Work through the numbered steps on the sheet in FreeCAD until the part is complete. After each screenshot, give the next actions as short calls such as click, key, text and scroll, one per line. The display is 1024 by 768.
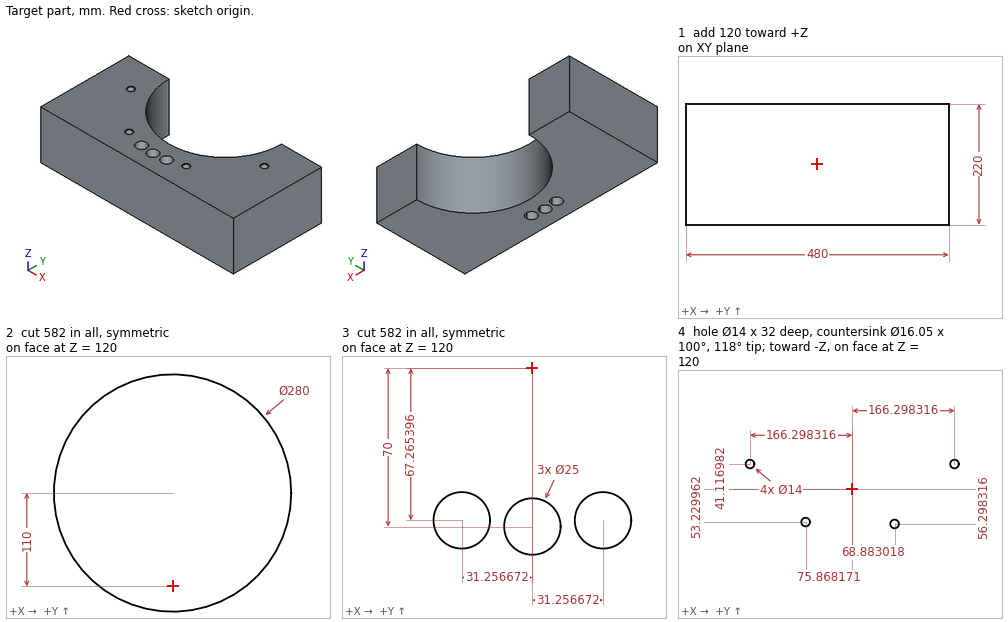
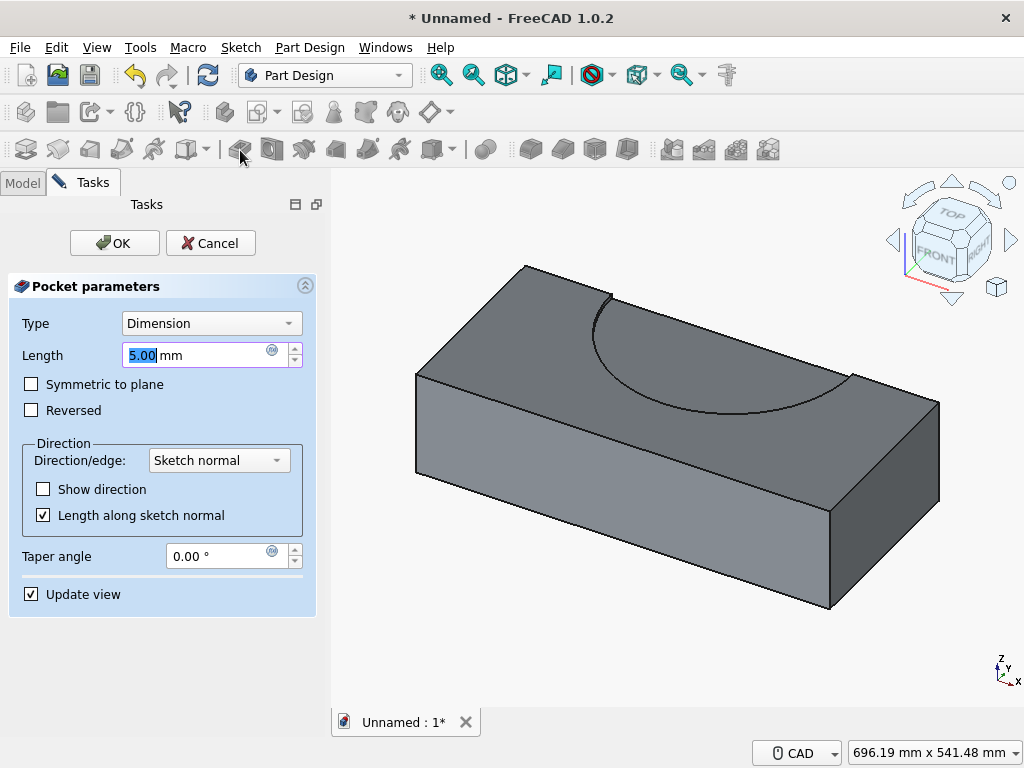
text(582)
key(Tab)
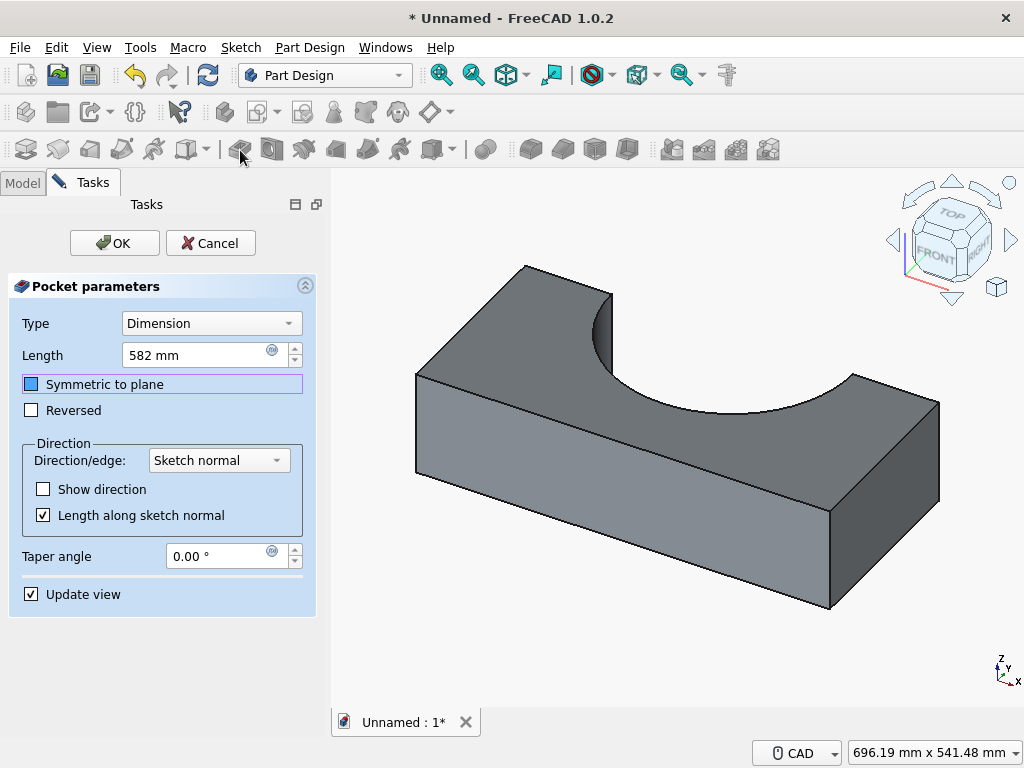
click(30, 384)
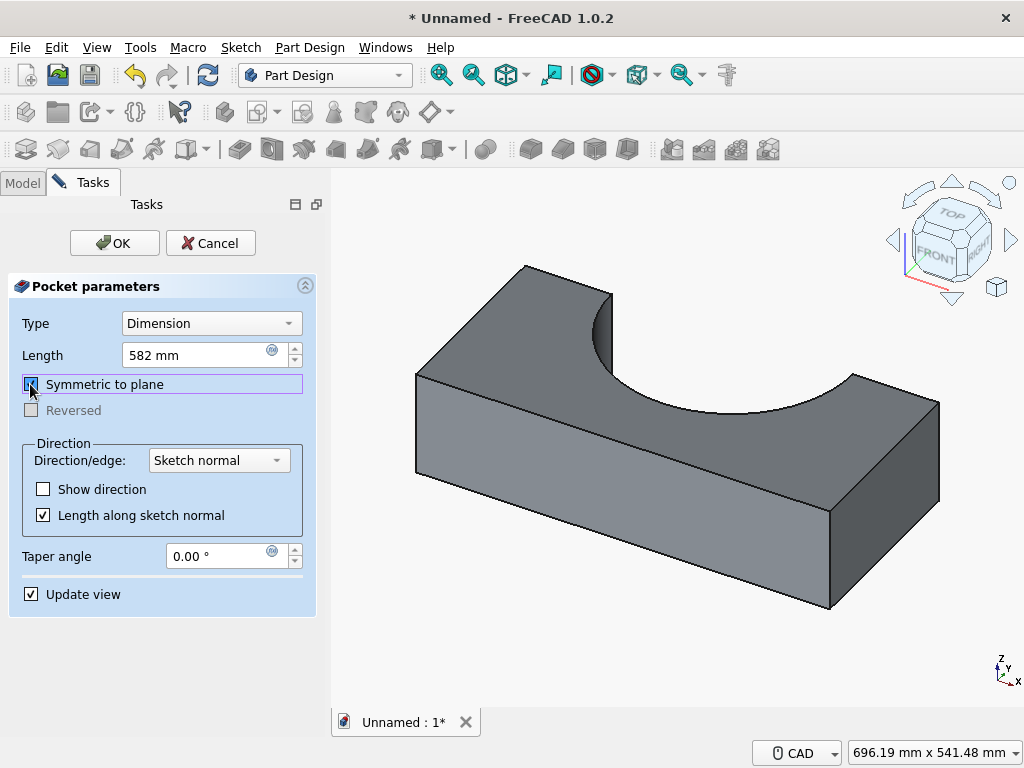
click(115, 243)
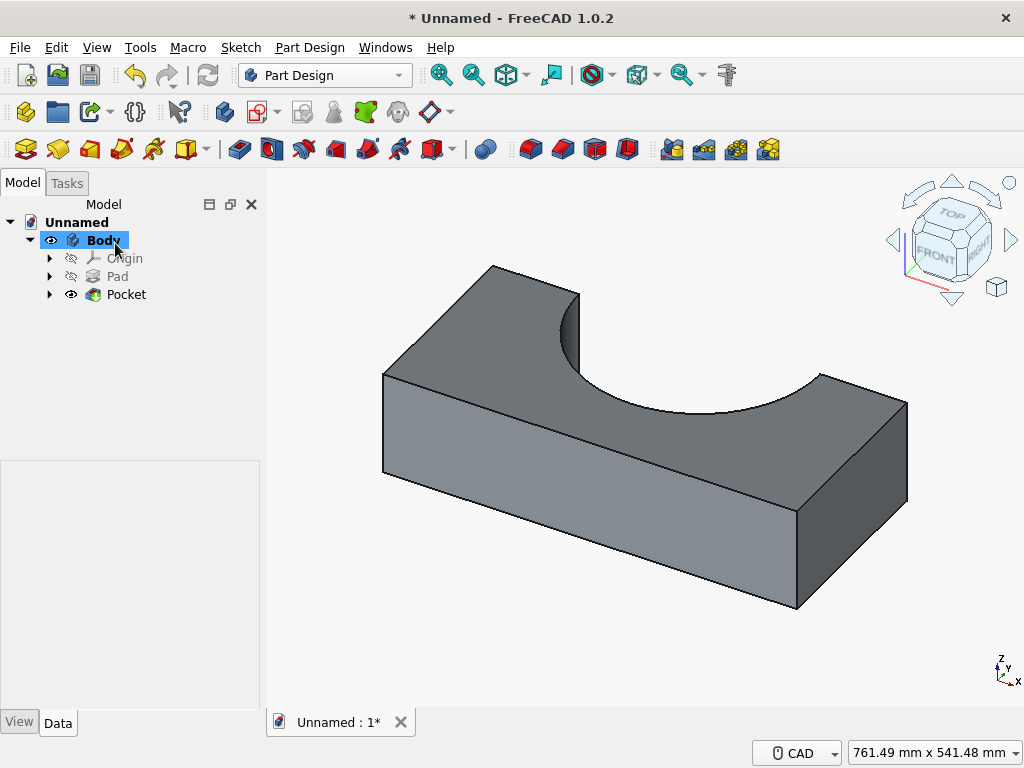
click(748, 442)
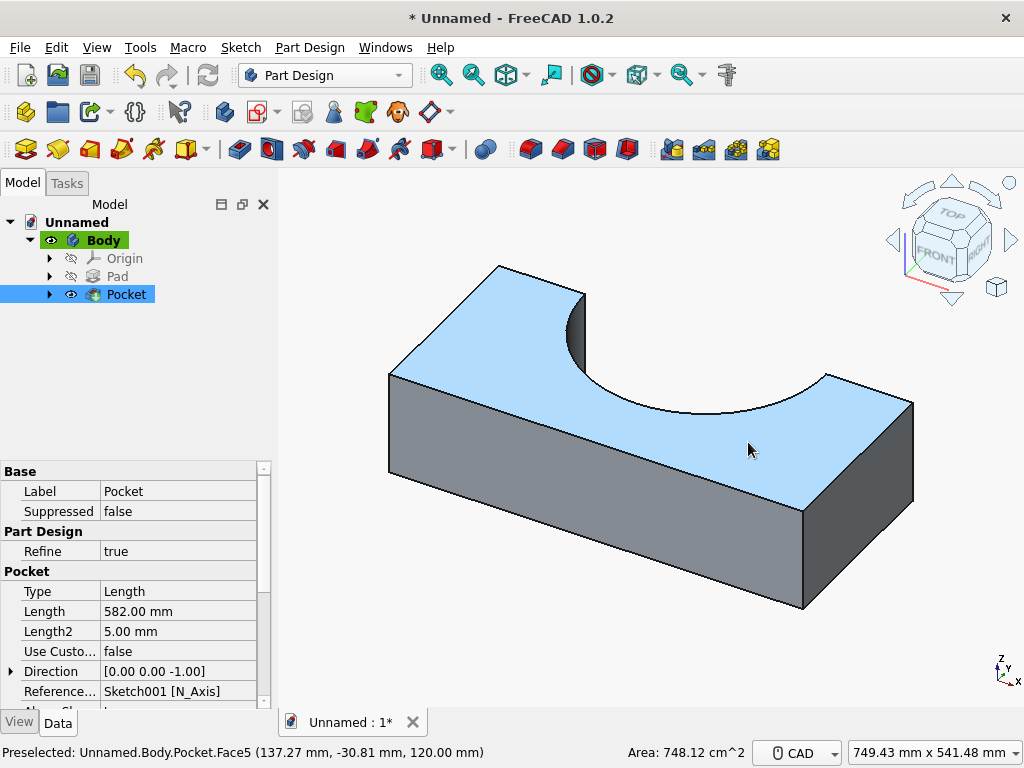
click(258, 112)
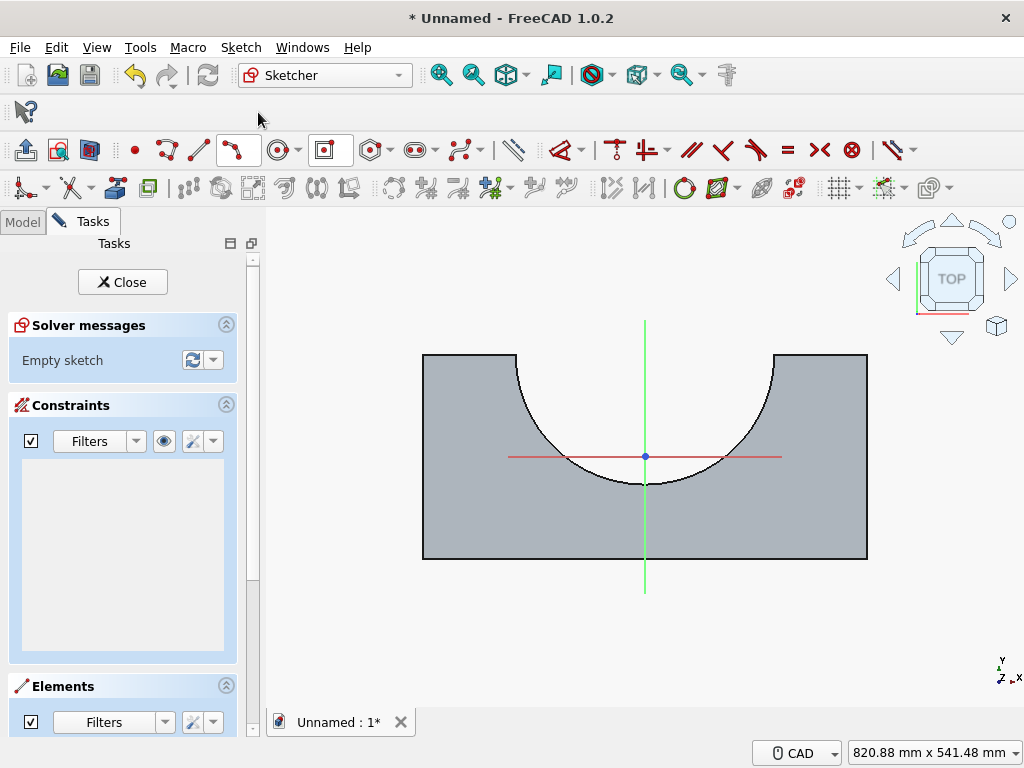
scroll(667, 508, up, 7)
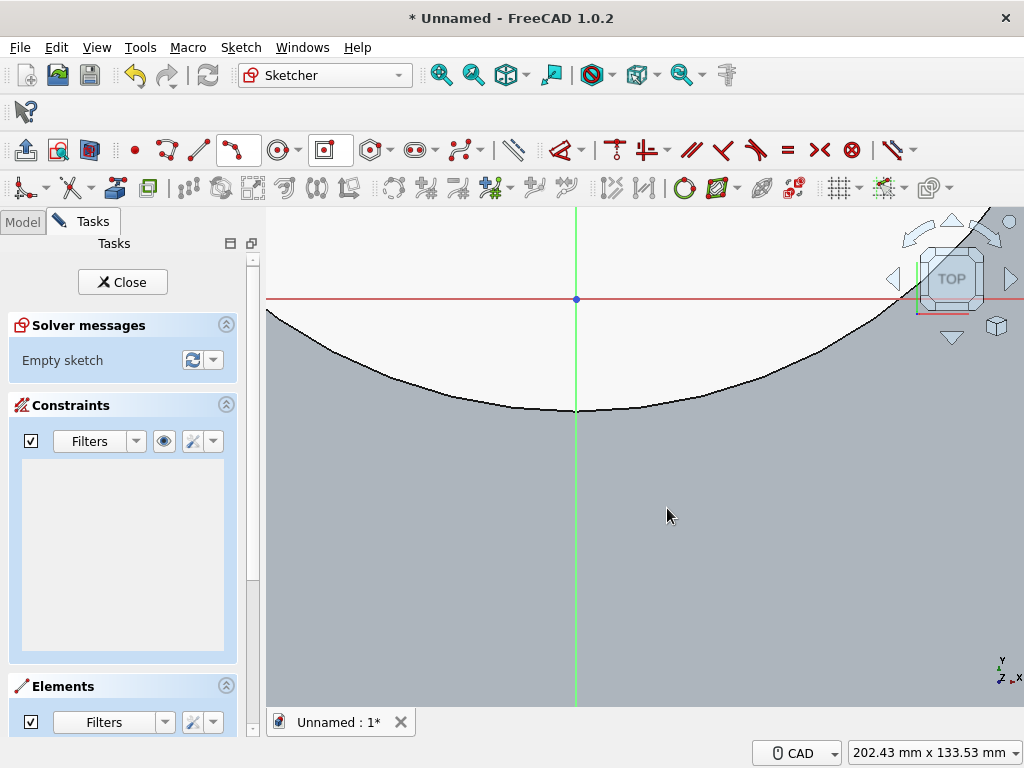
key(g)
key(c)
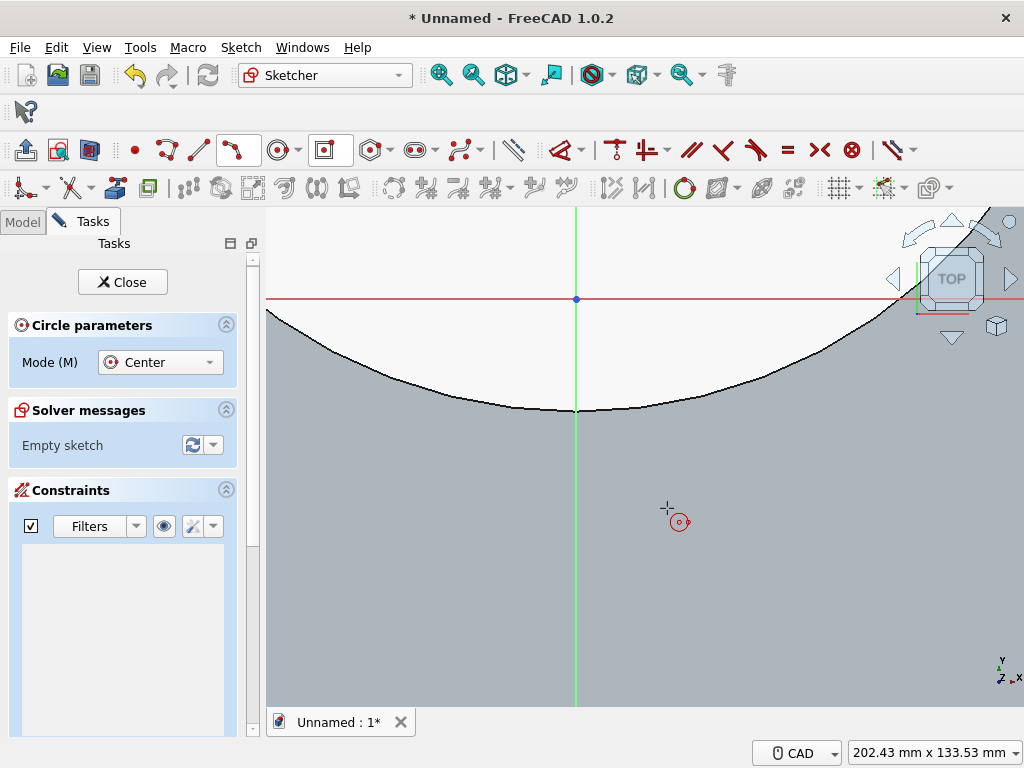
click(576, 561)
move(609, 528)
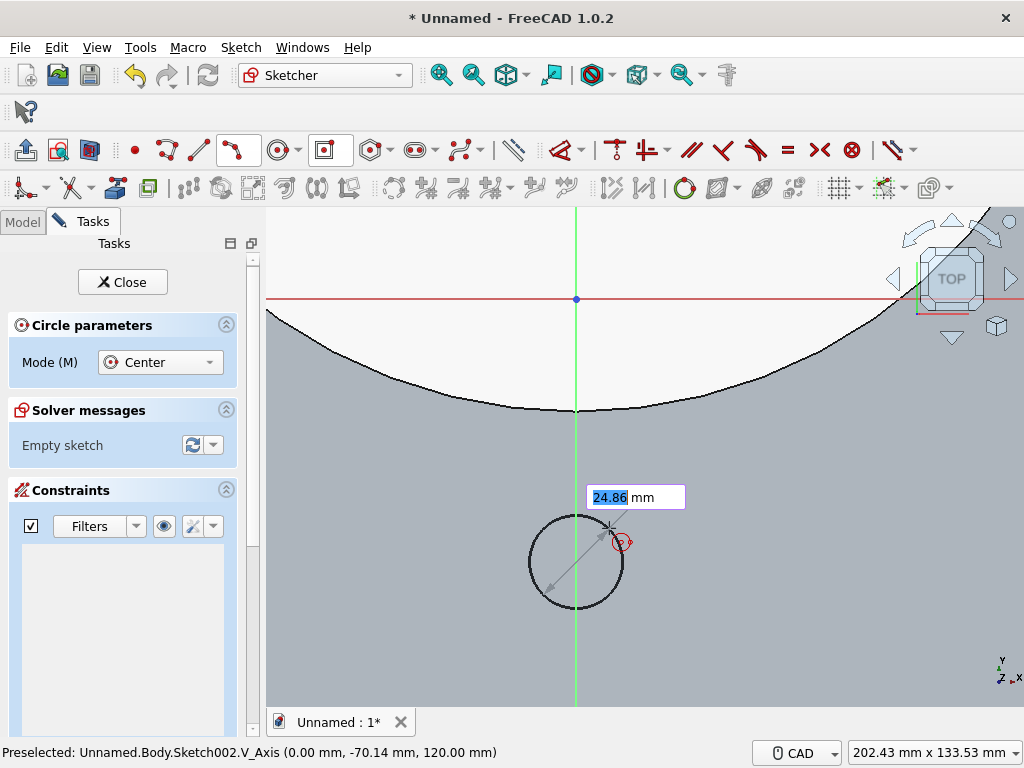
text(25)
key(Return)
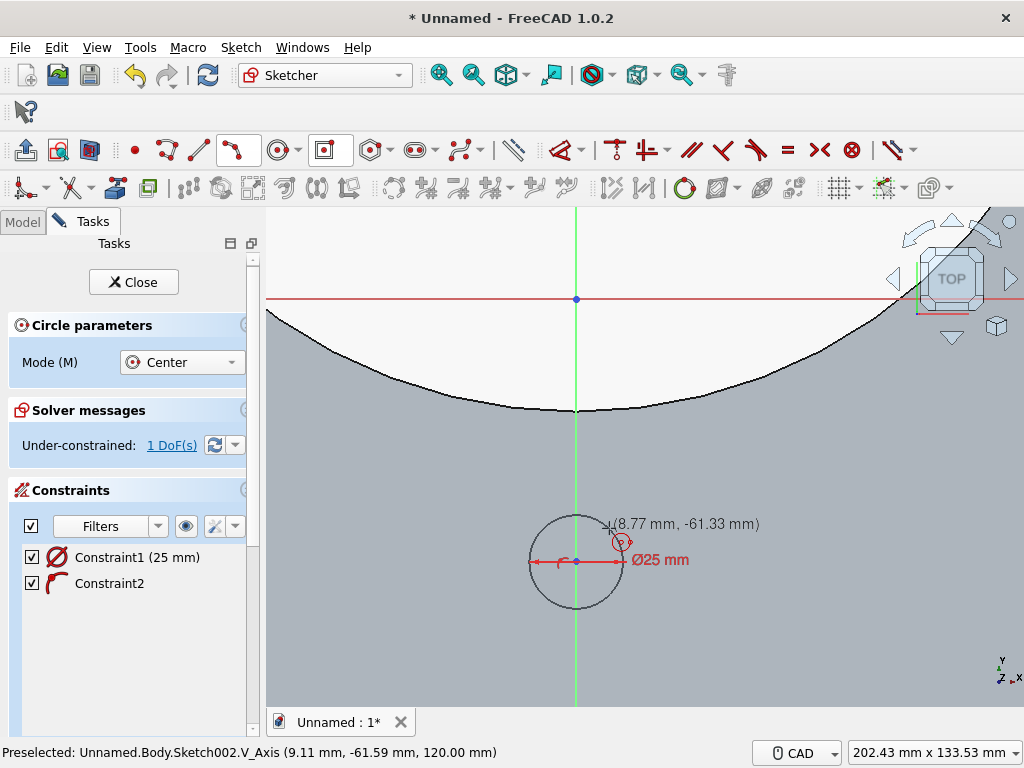
click(459, 551)
move(492, 518)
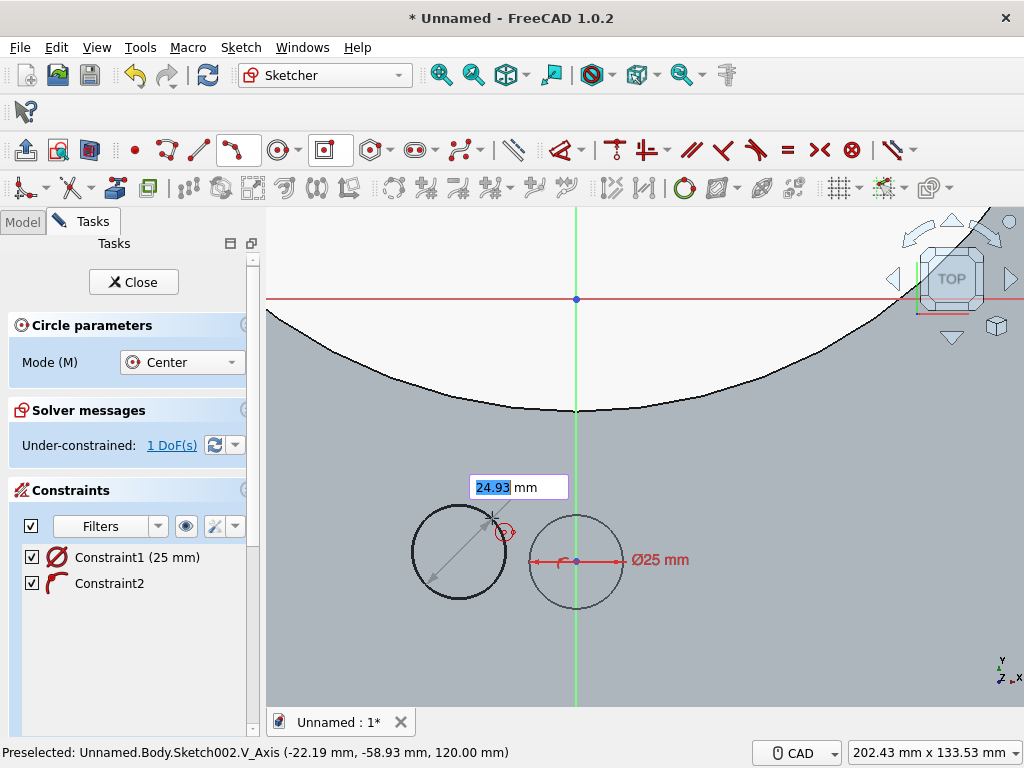
text(25)
key(Return)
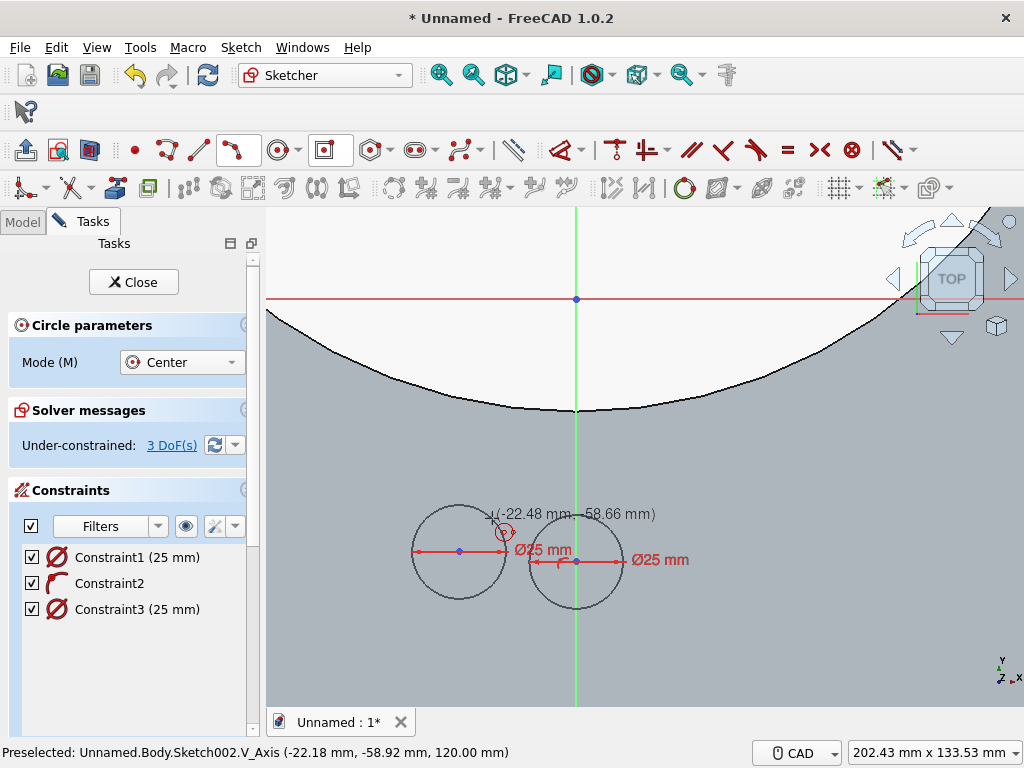
click(693, 551)
move(726, 518)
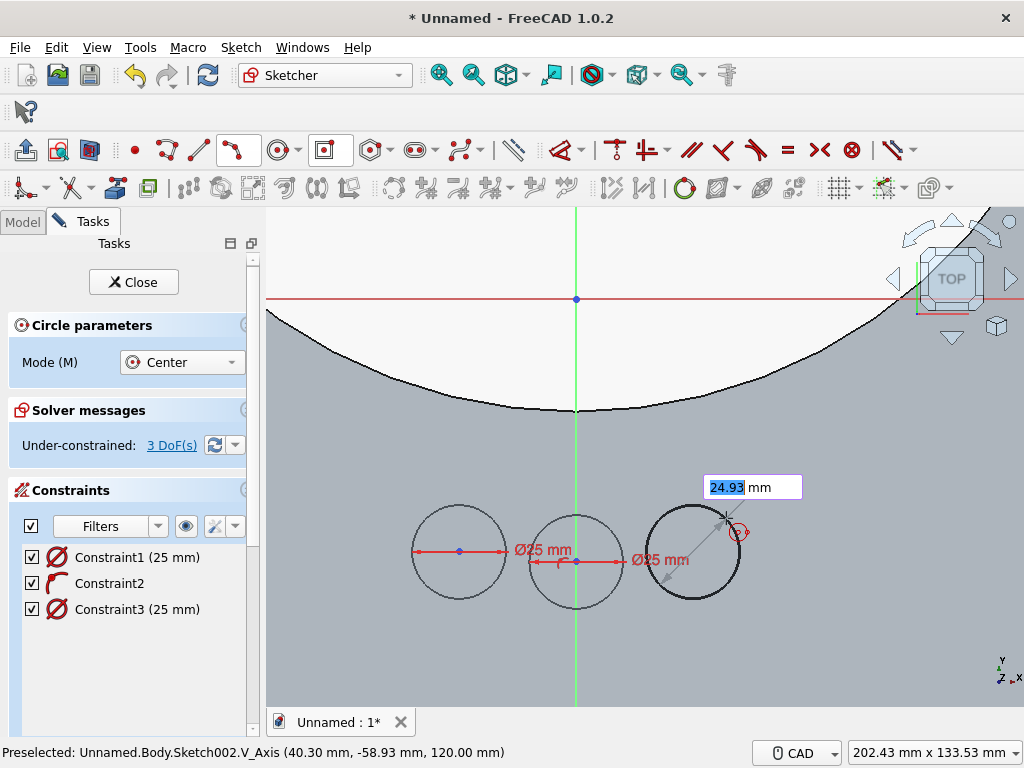
text(25)
key(Return)
key(Escape)